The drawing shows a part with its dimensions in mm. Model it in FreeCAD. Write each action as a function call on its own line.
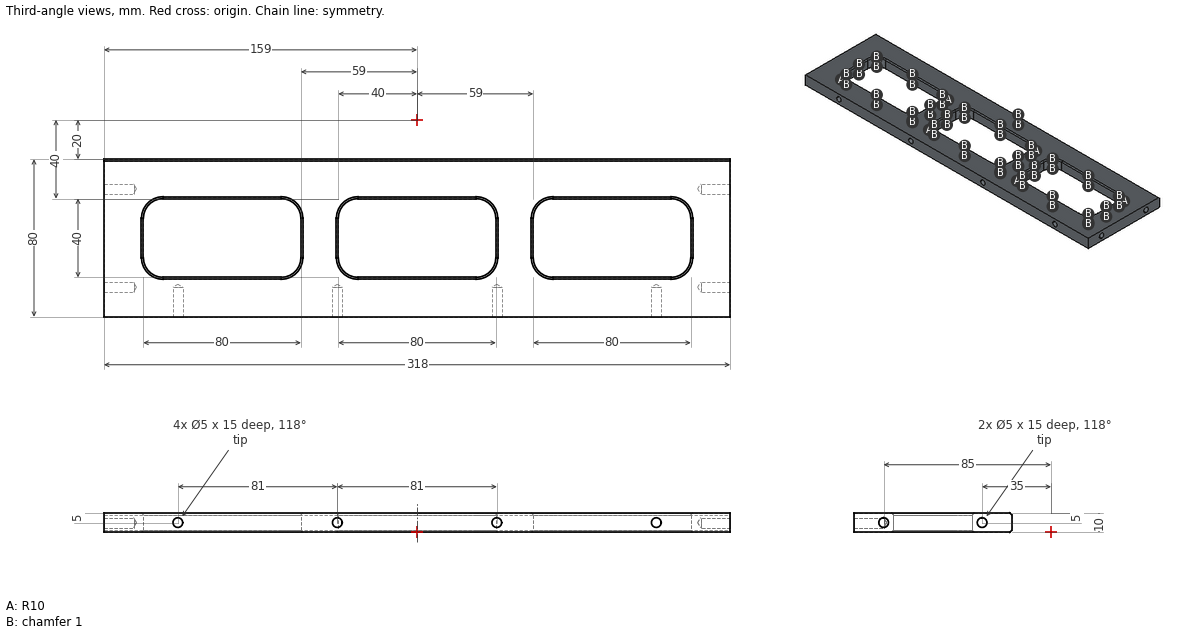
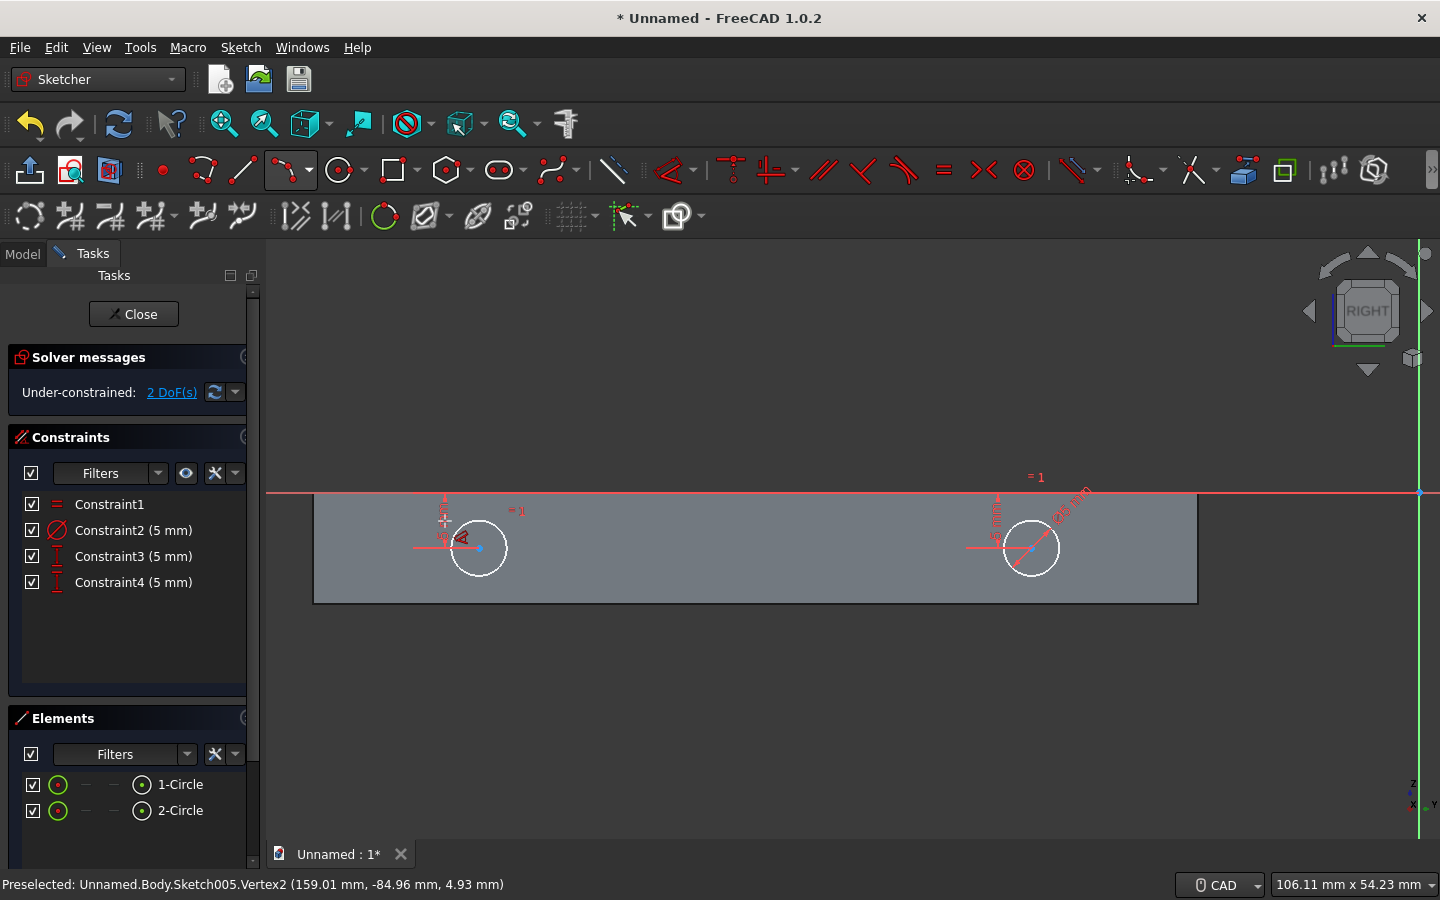
click(1032, 548)
click(1153, 459)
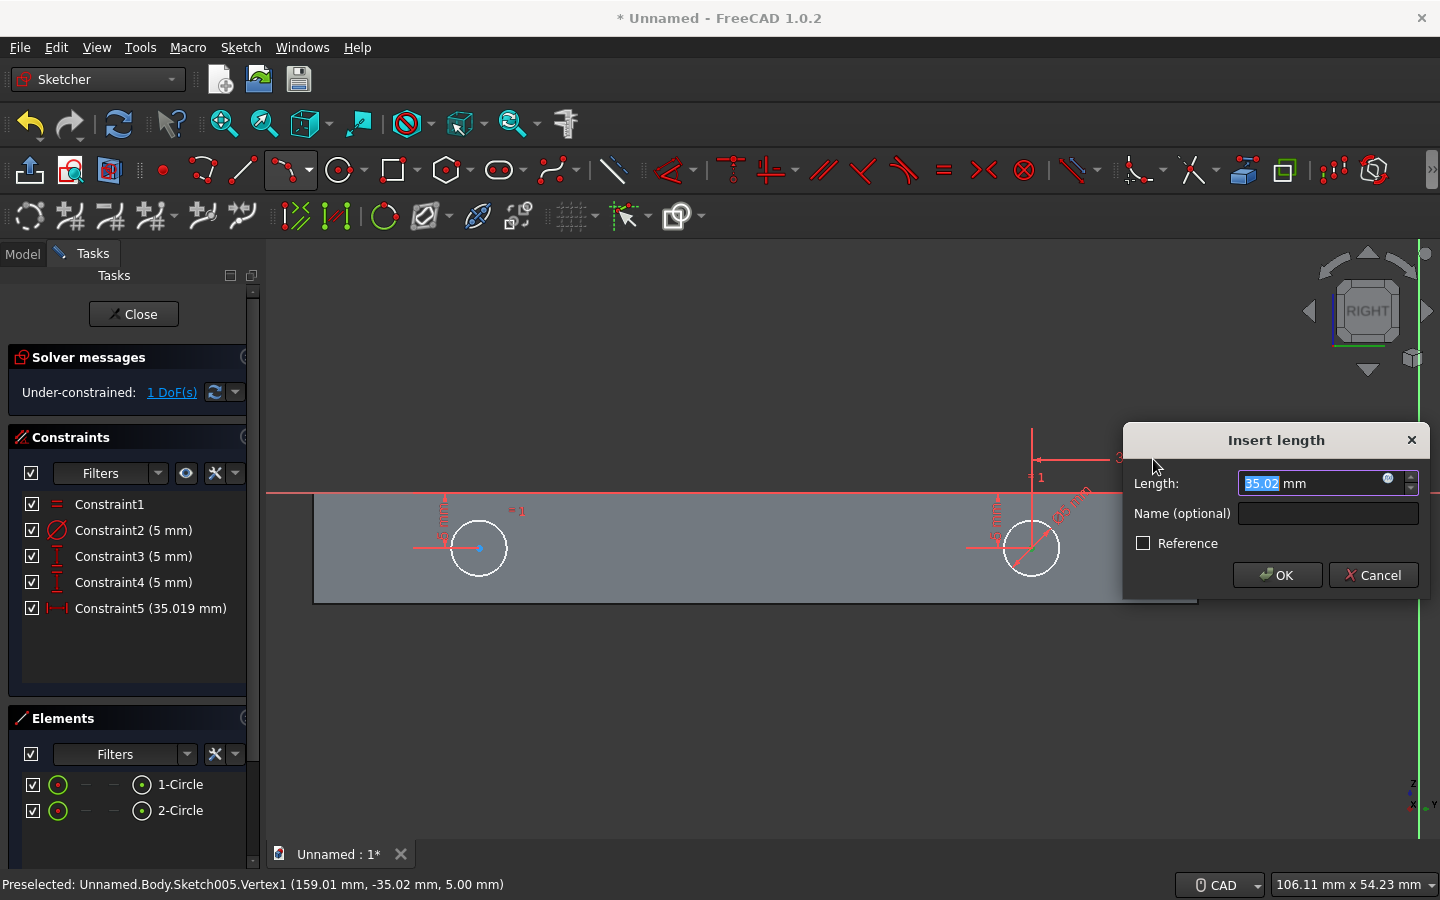
text(35)
key(Return)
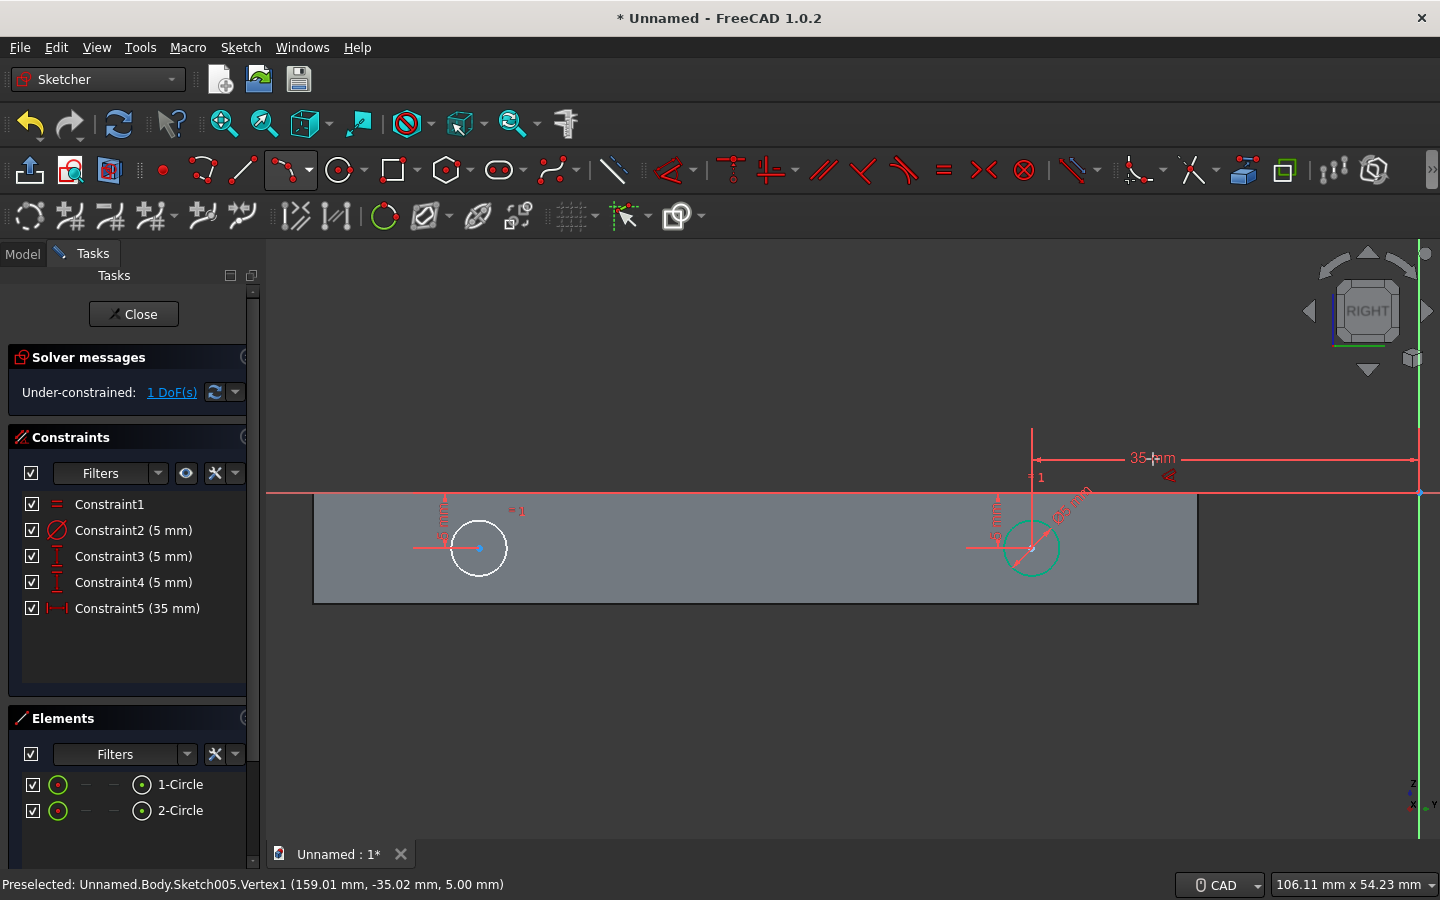
click(479, 548)
click(877, 459)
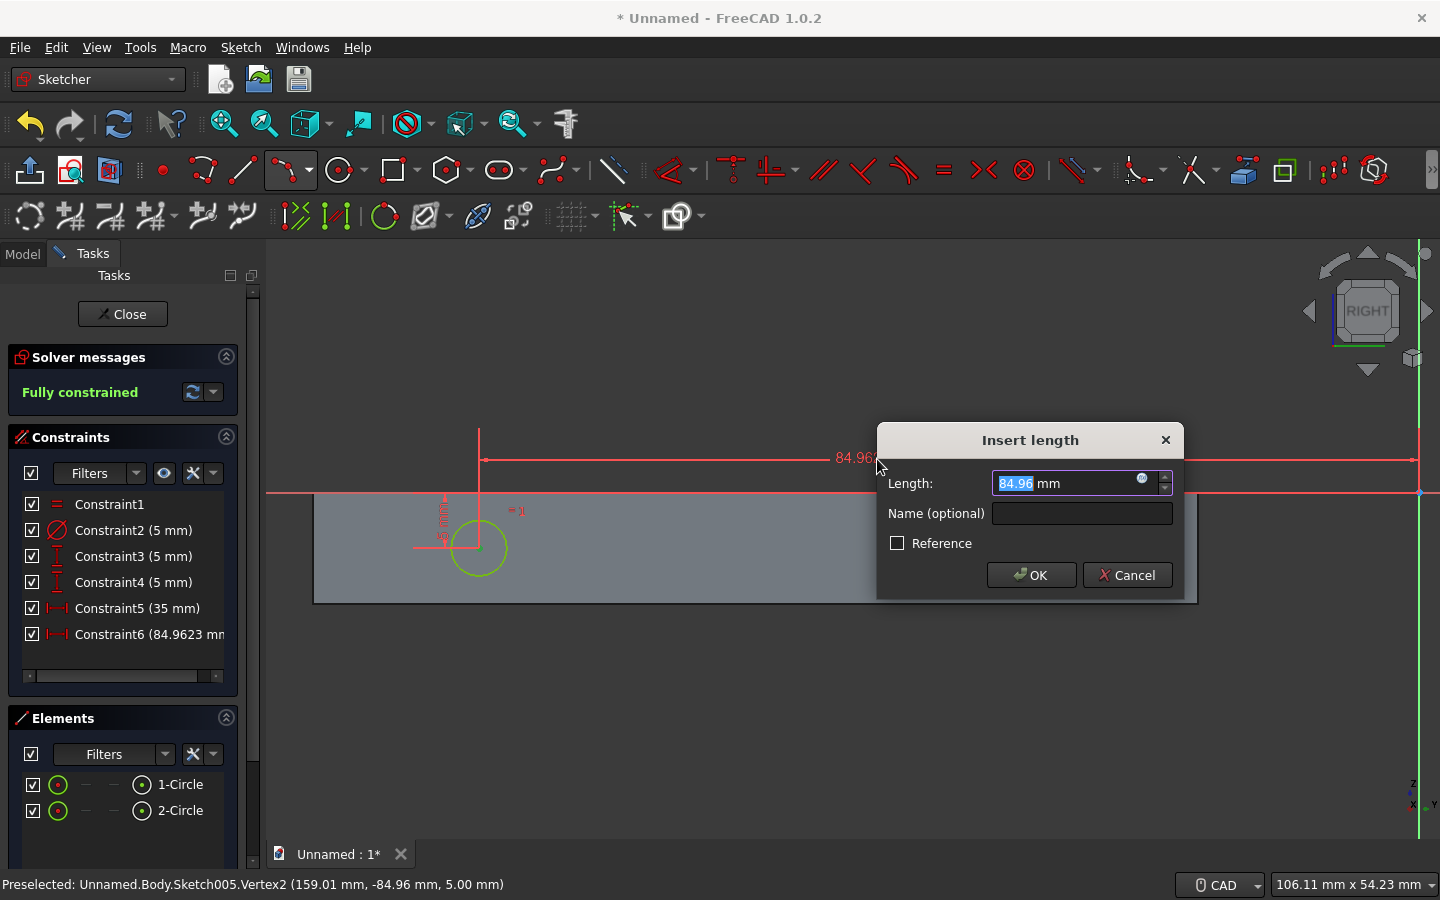
text(85)
key(Return)
key(Escape)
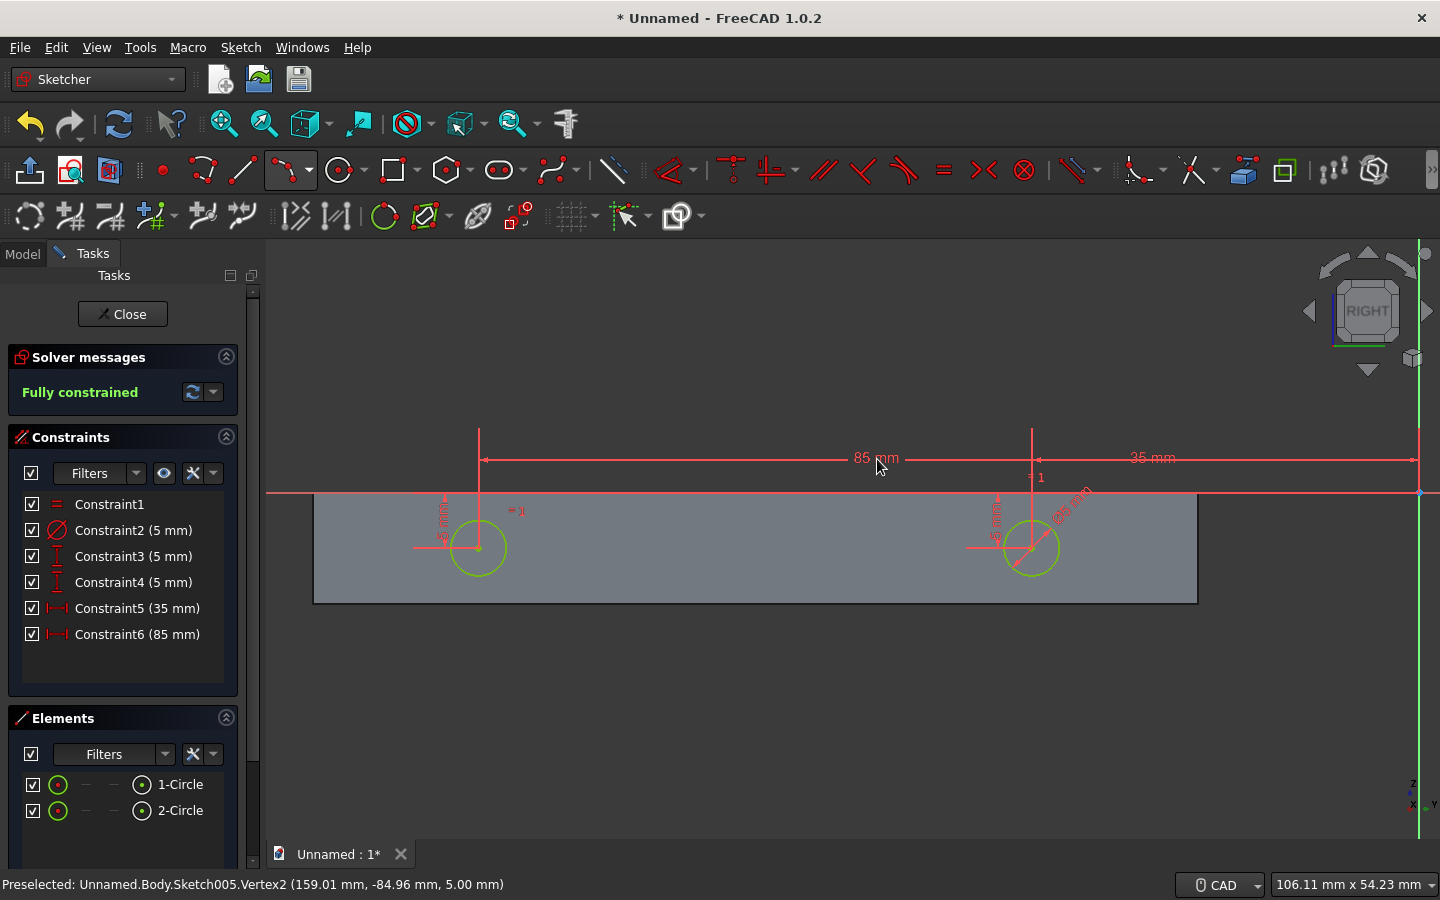
click(123, 314)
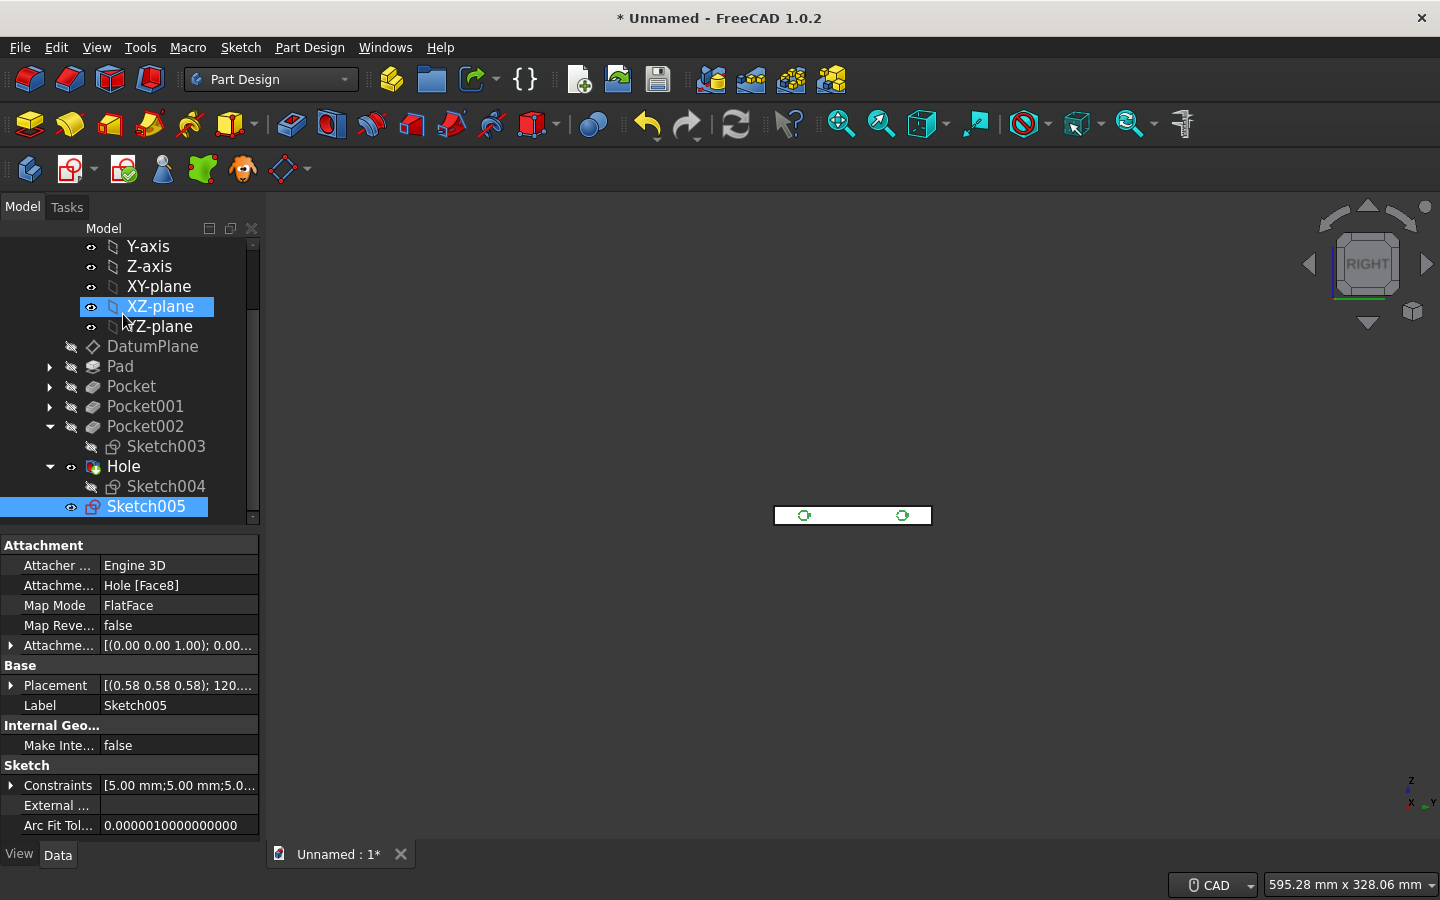
click(332, 124)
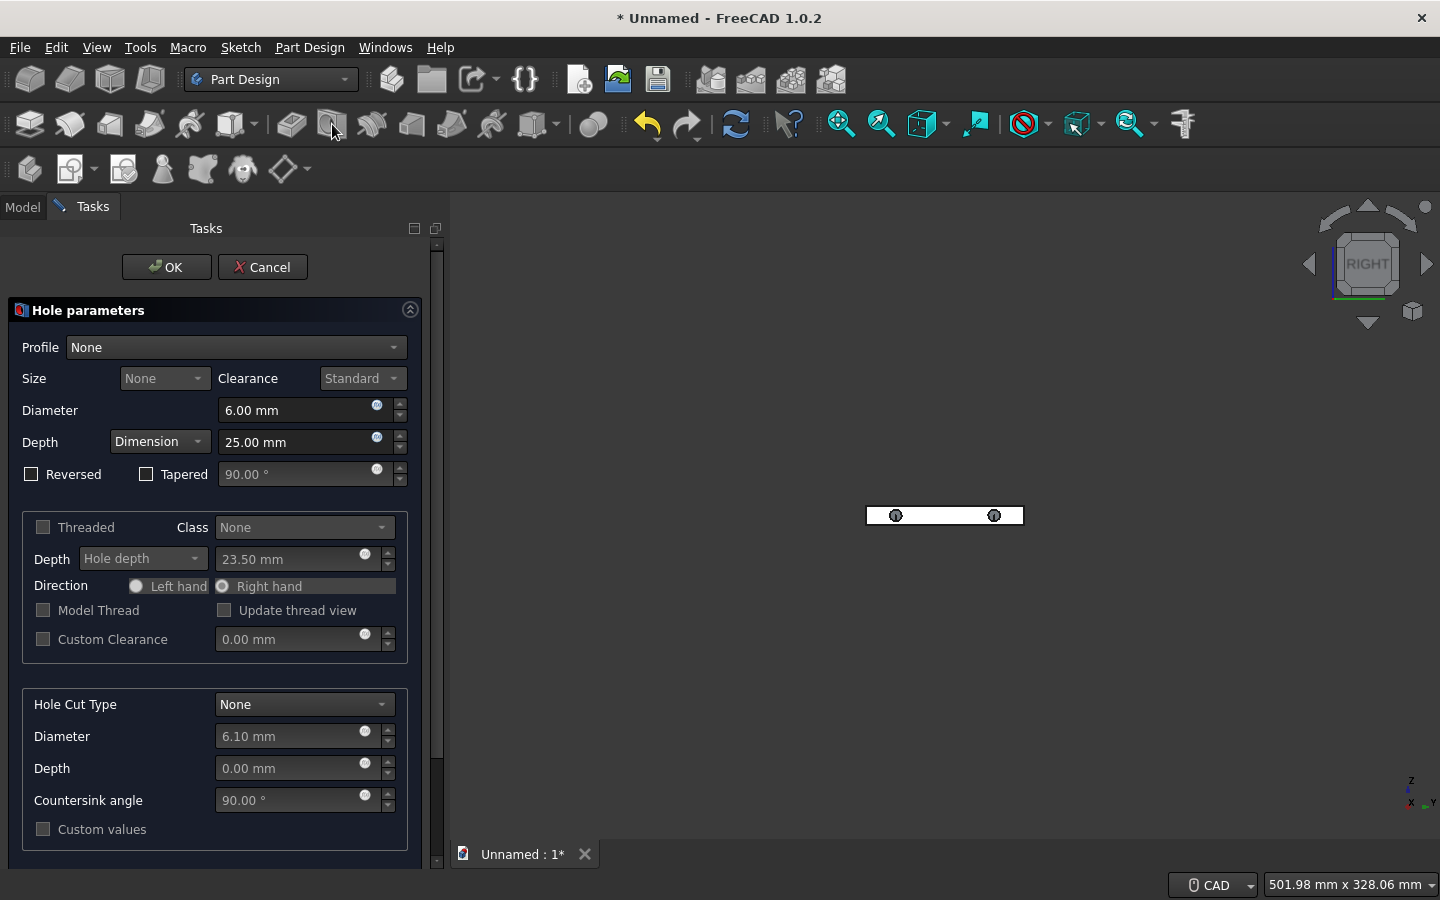
triple_click(305, 410)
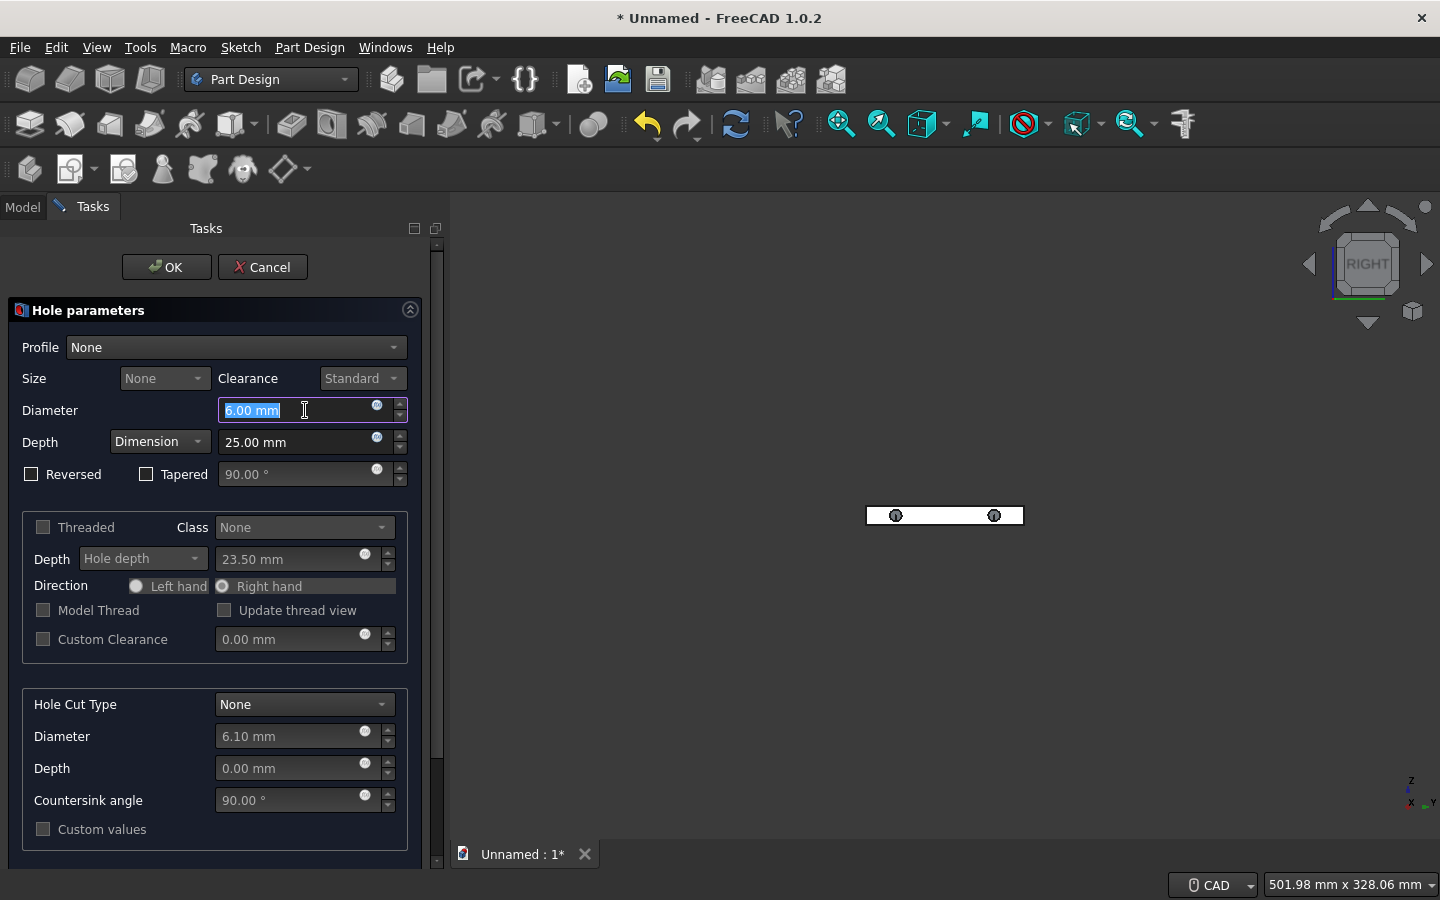
text(5)
key(Tab)